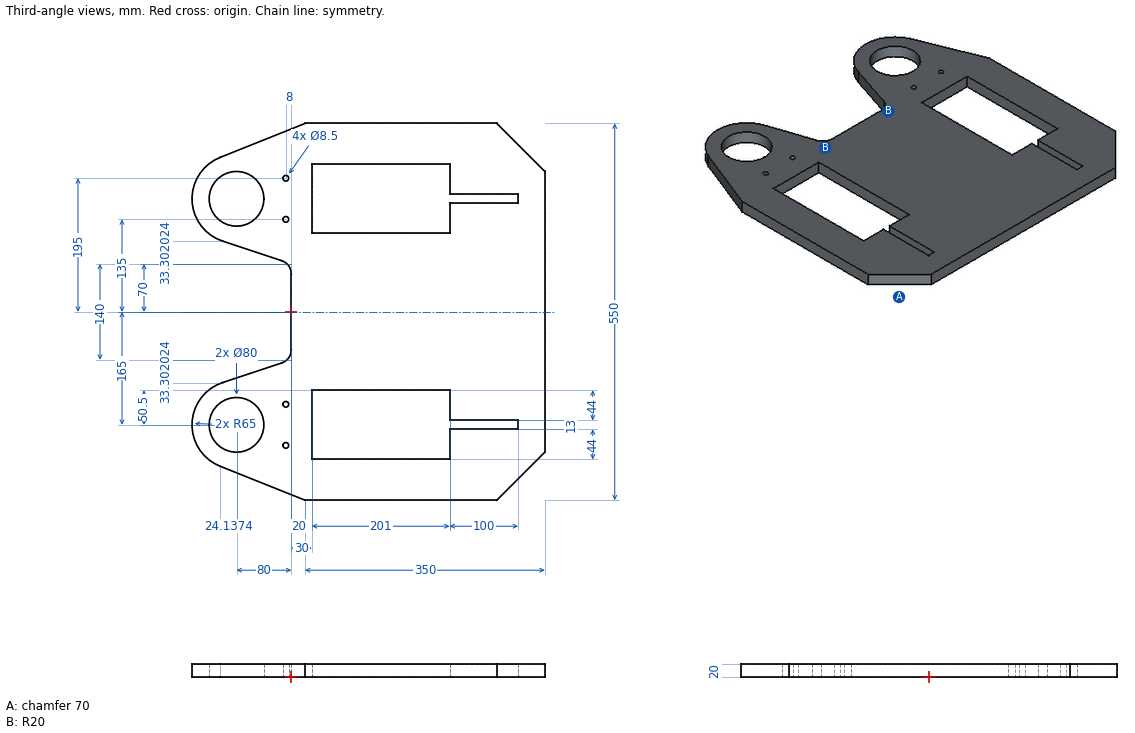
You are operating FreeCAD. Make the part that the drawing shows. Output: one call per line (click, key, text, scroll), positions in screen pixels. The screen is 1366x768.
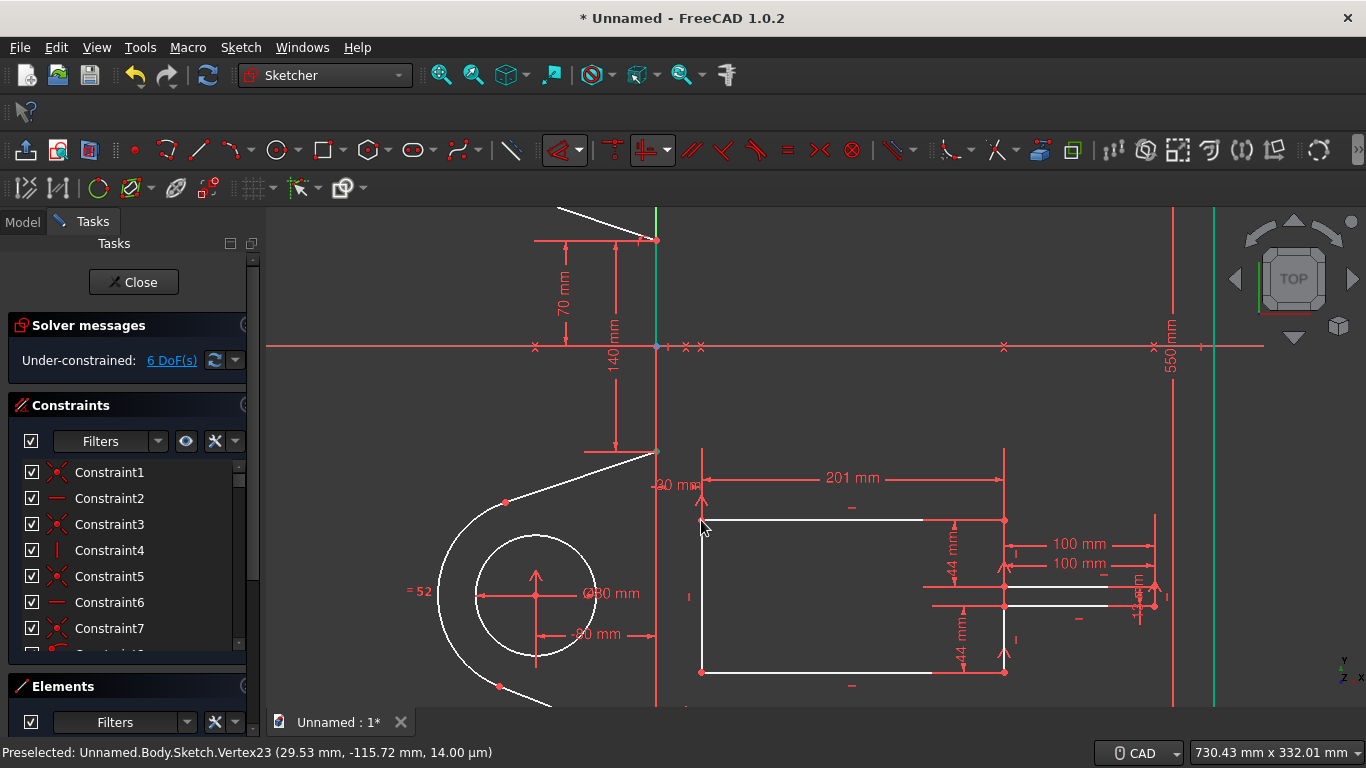
click(536, 596)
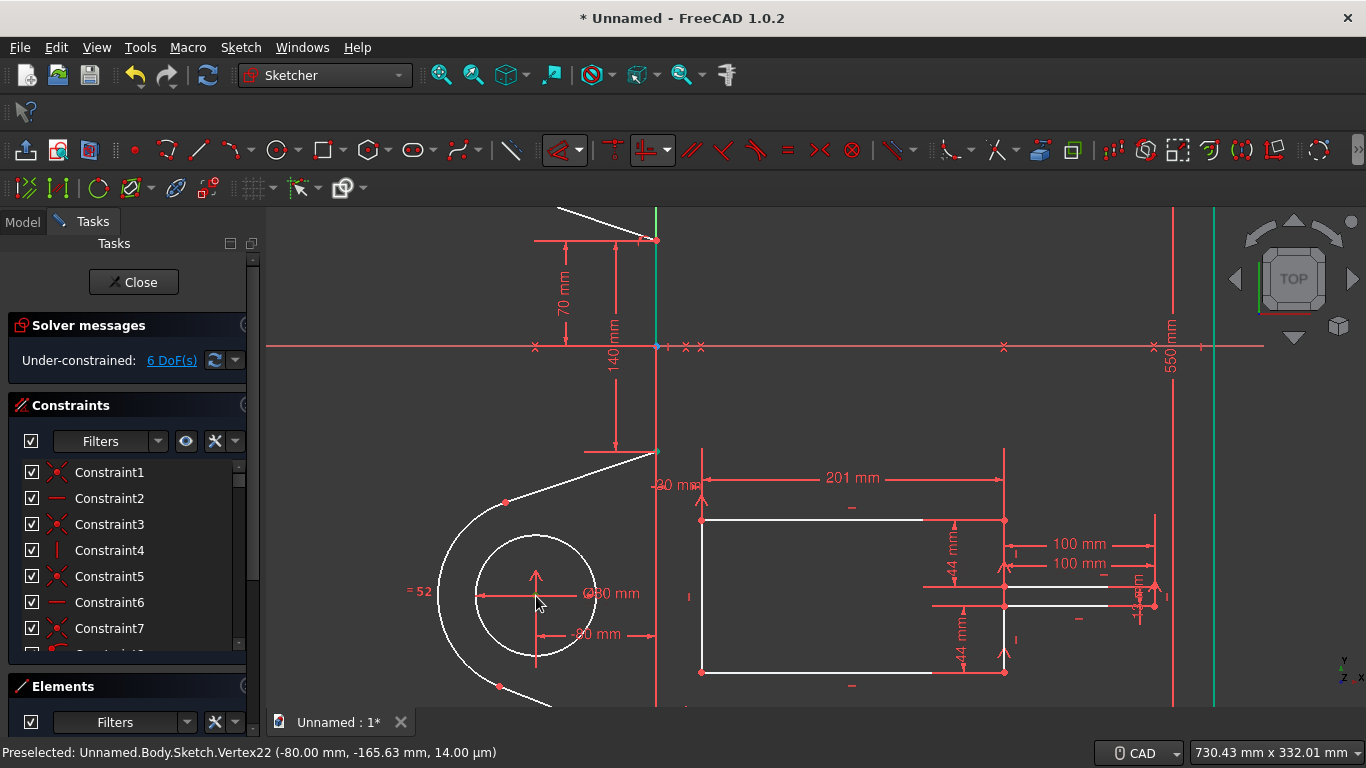
key(i)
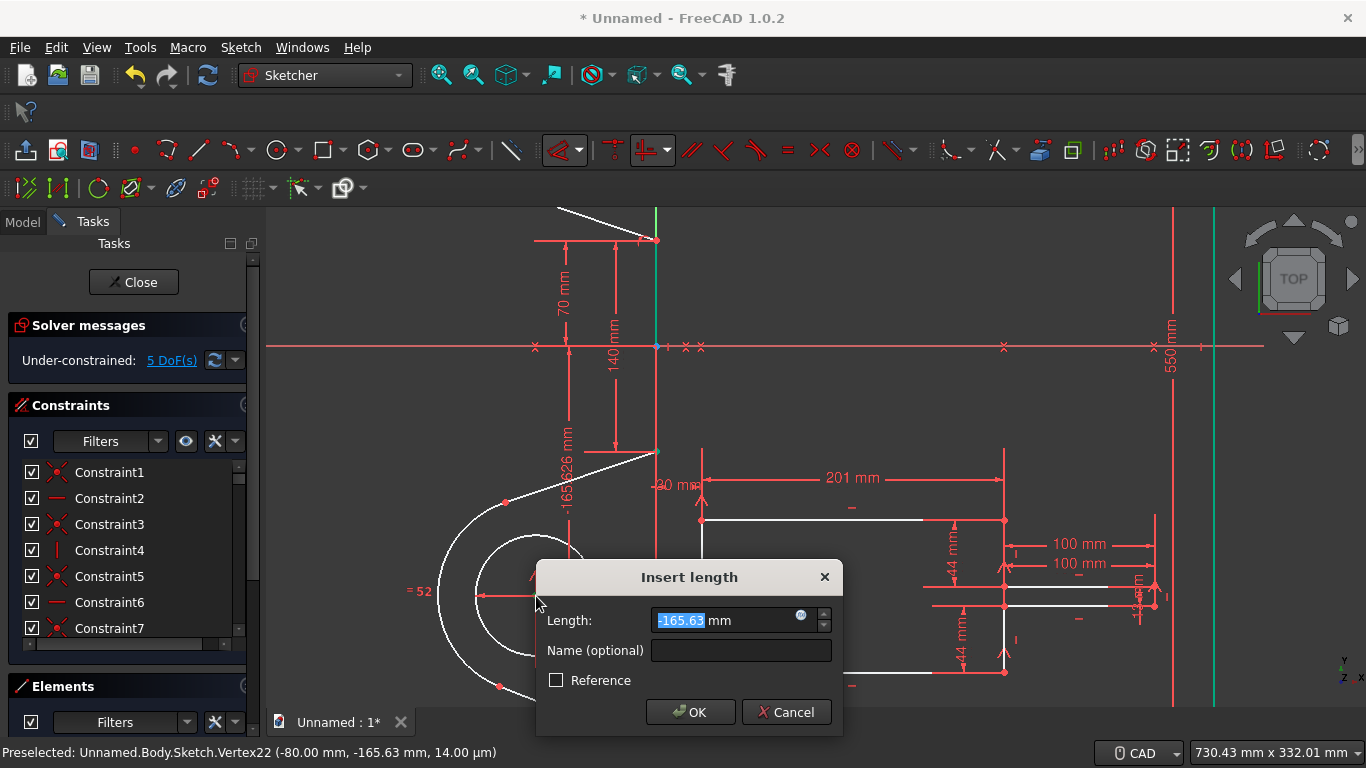
text(-165)
key(Return)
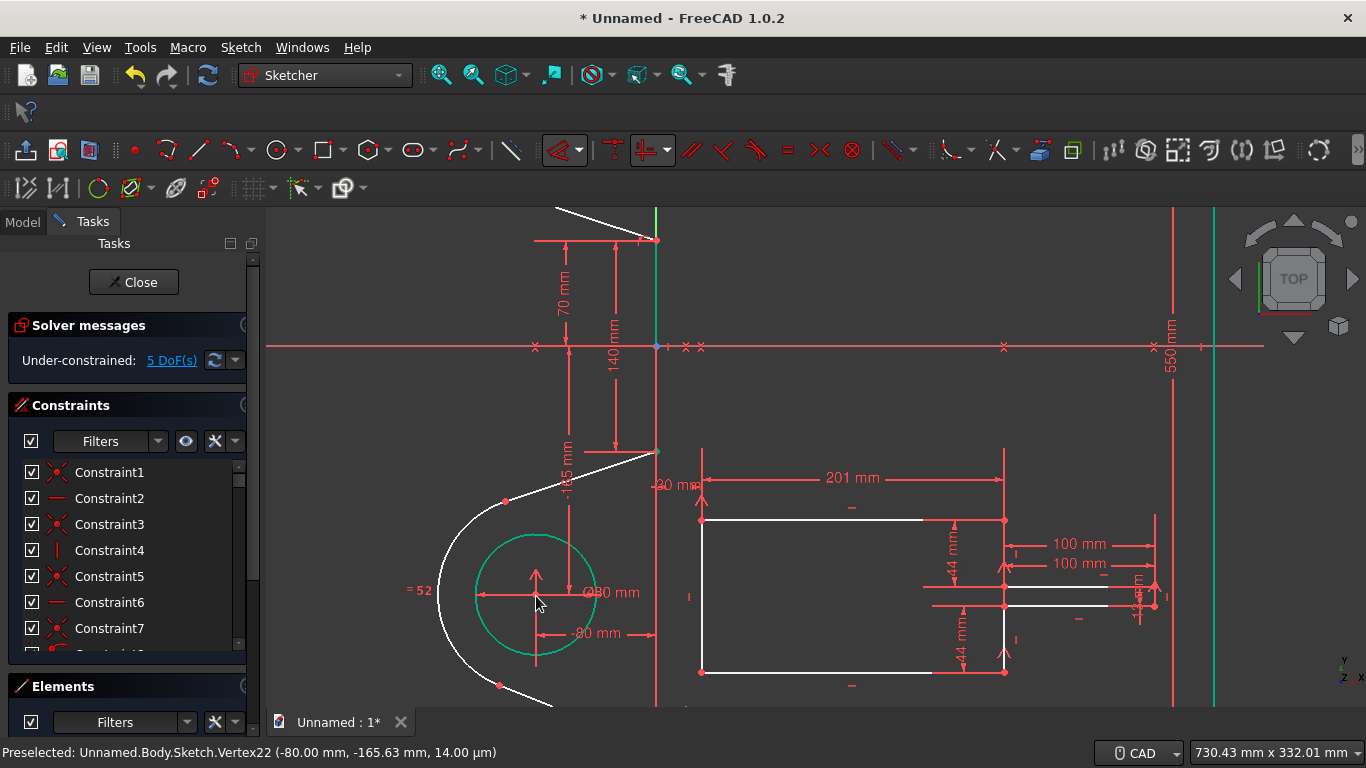
click(702, 520)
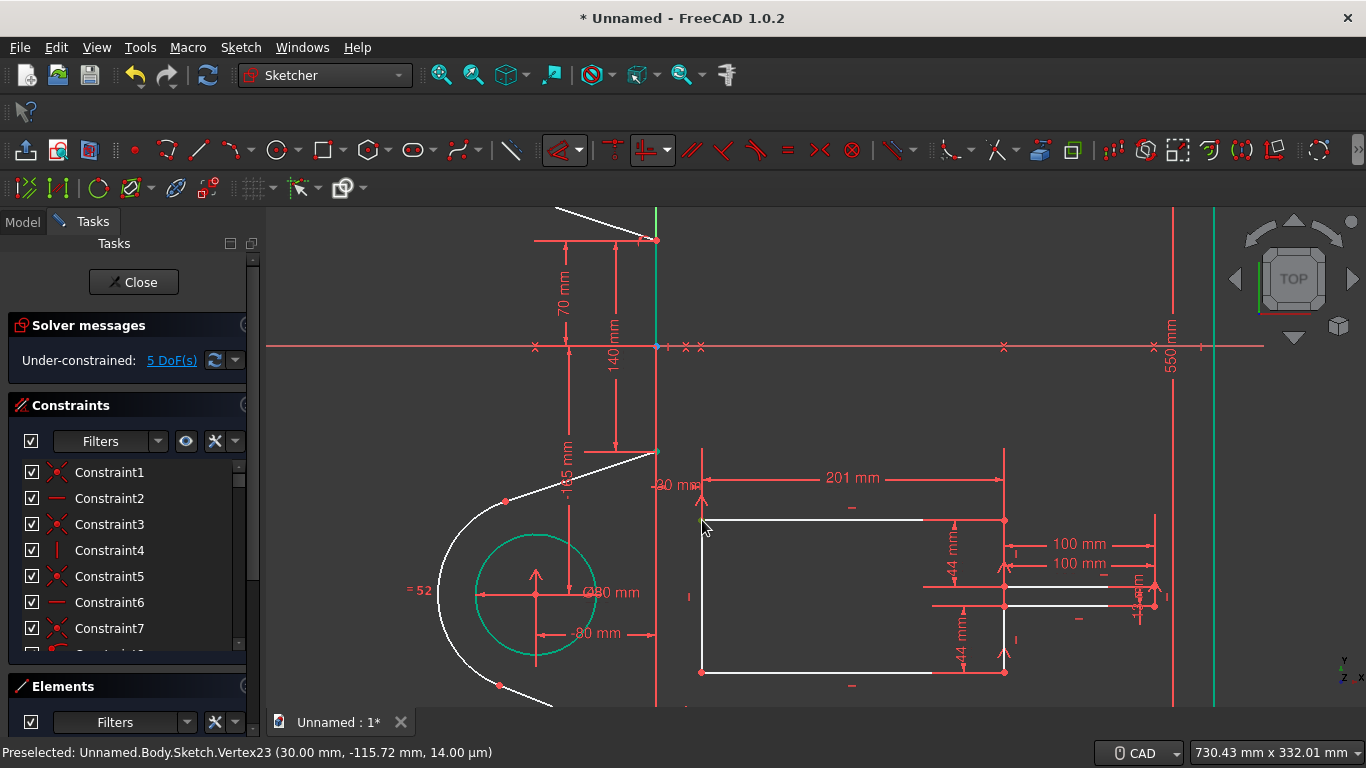
click(536, 595)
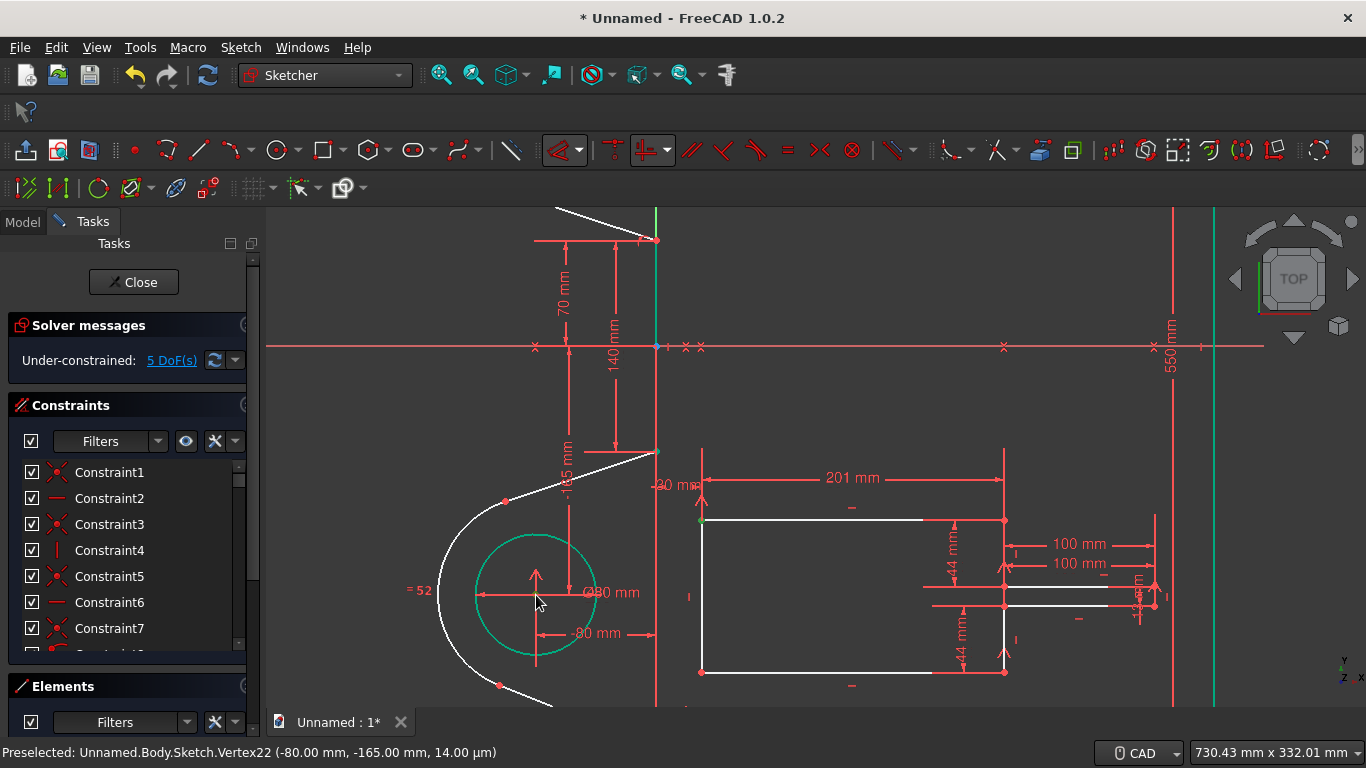
key(i)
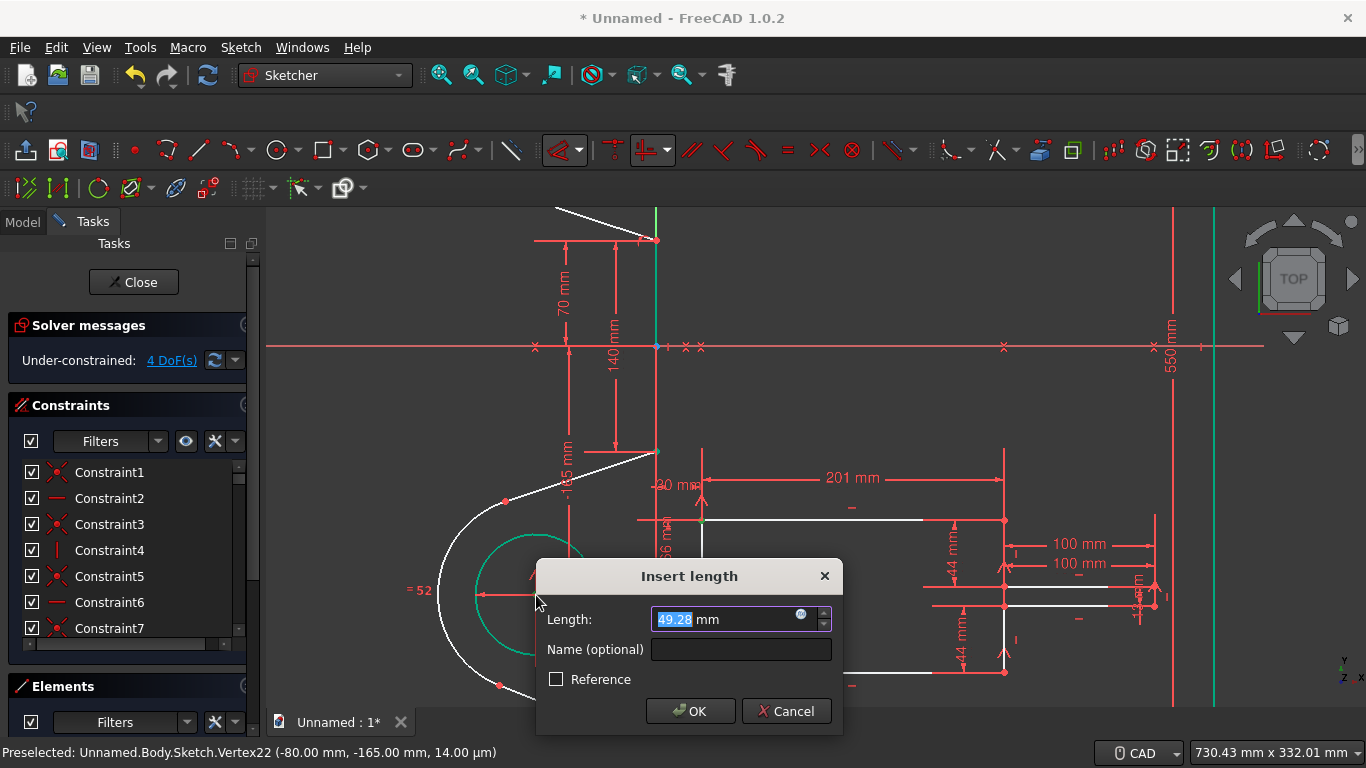
text(50.5)
key(Return)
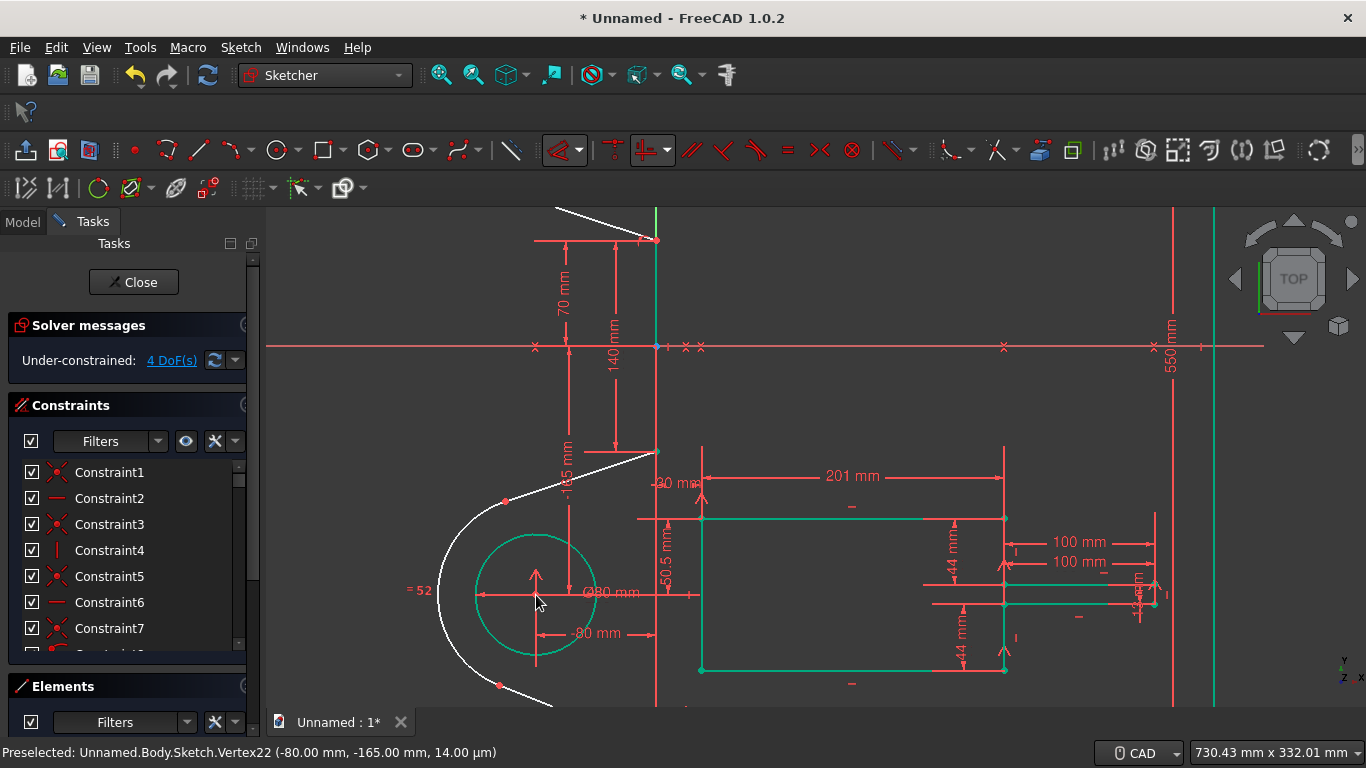
scroll(702, 522, down, 5)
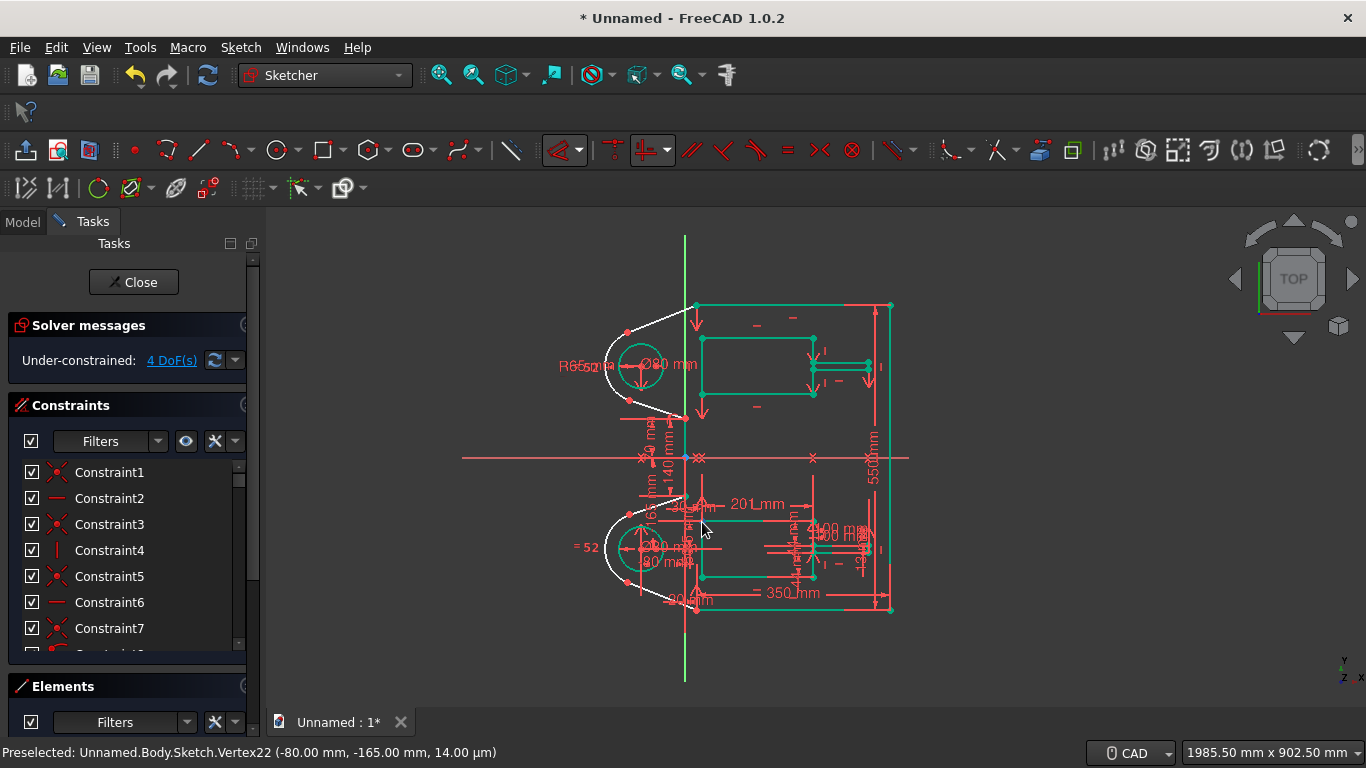
scroll(628, 583, up, 6)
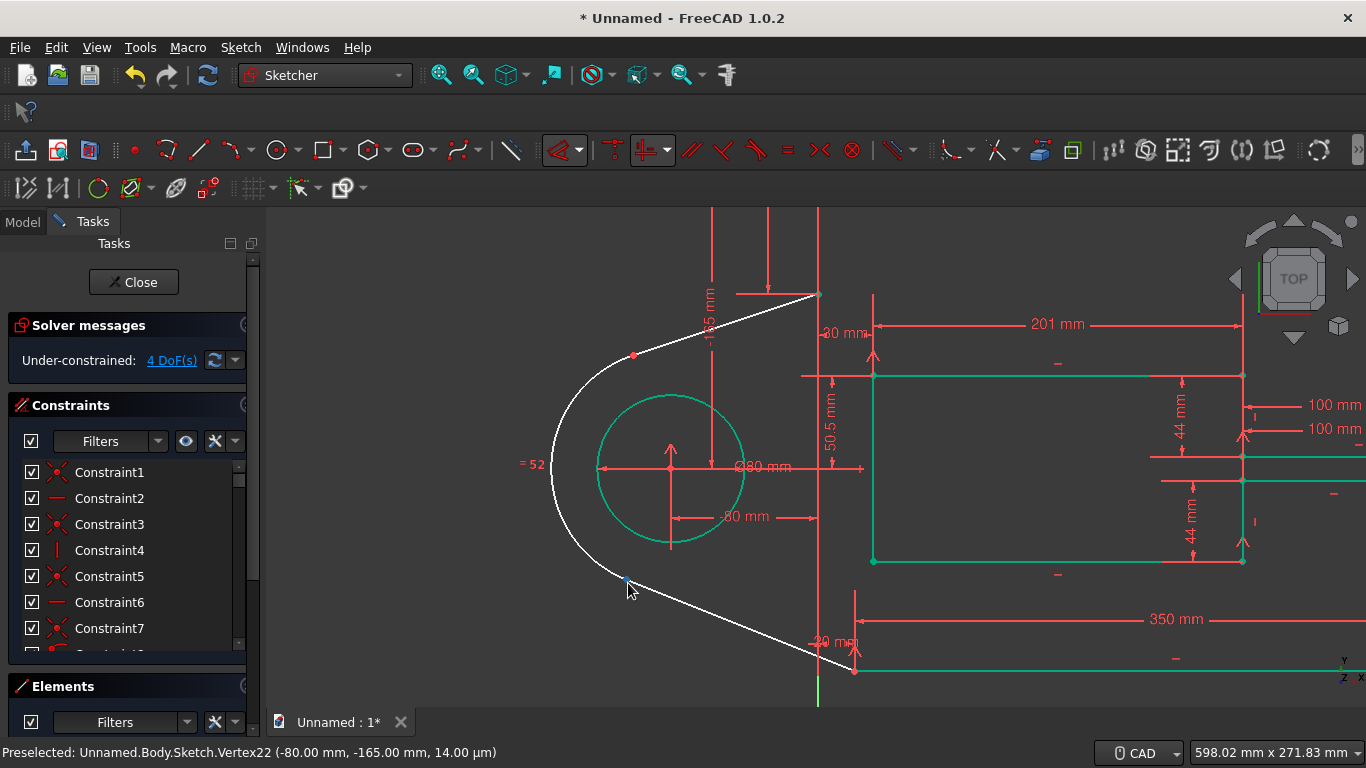
click(627, 580)